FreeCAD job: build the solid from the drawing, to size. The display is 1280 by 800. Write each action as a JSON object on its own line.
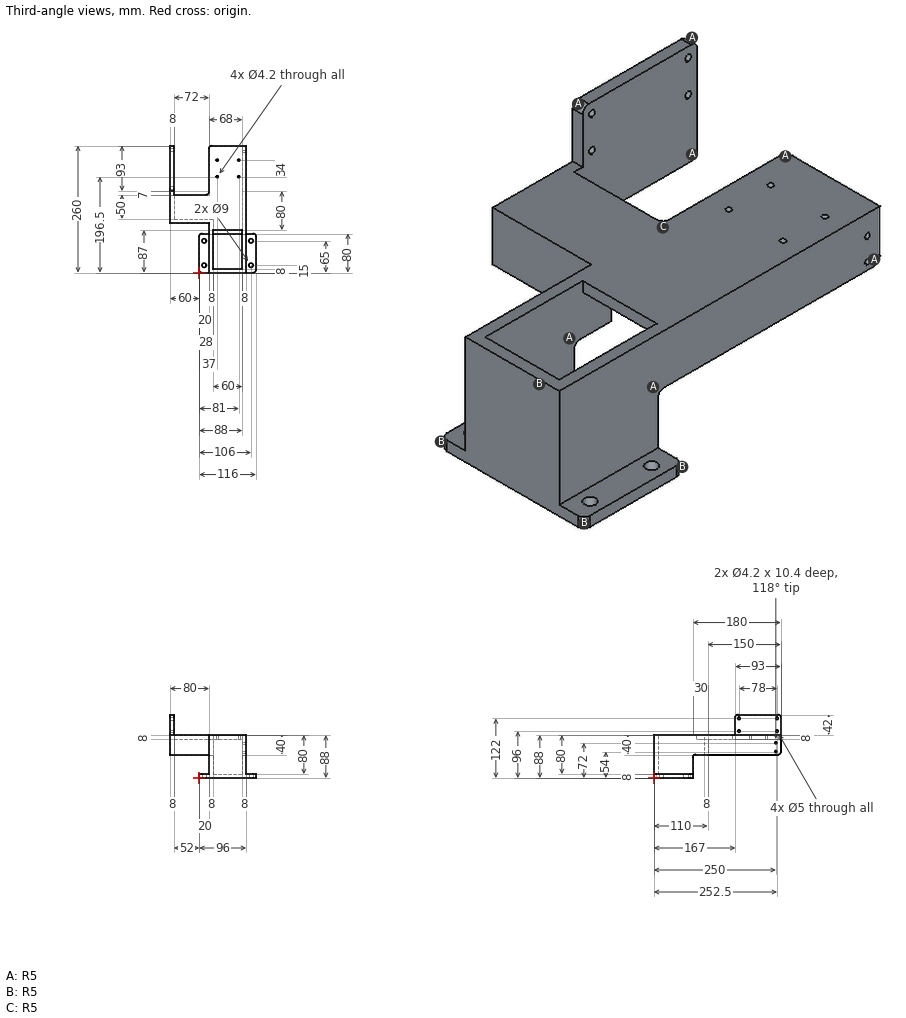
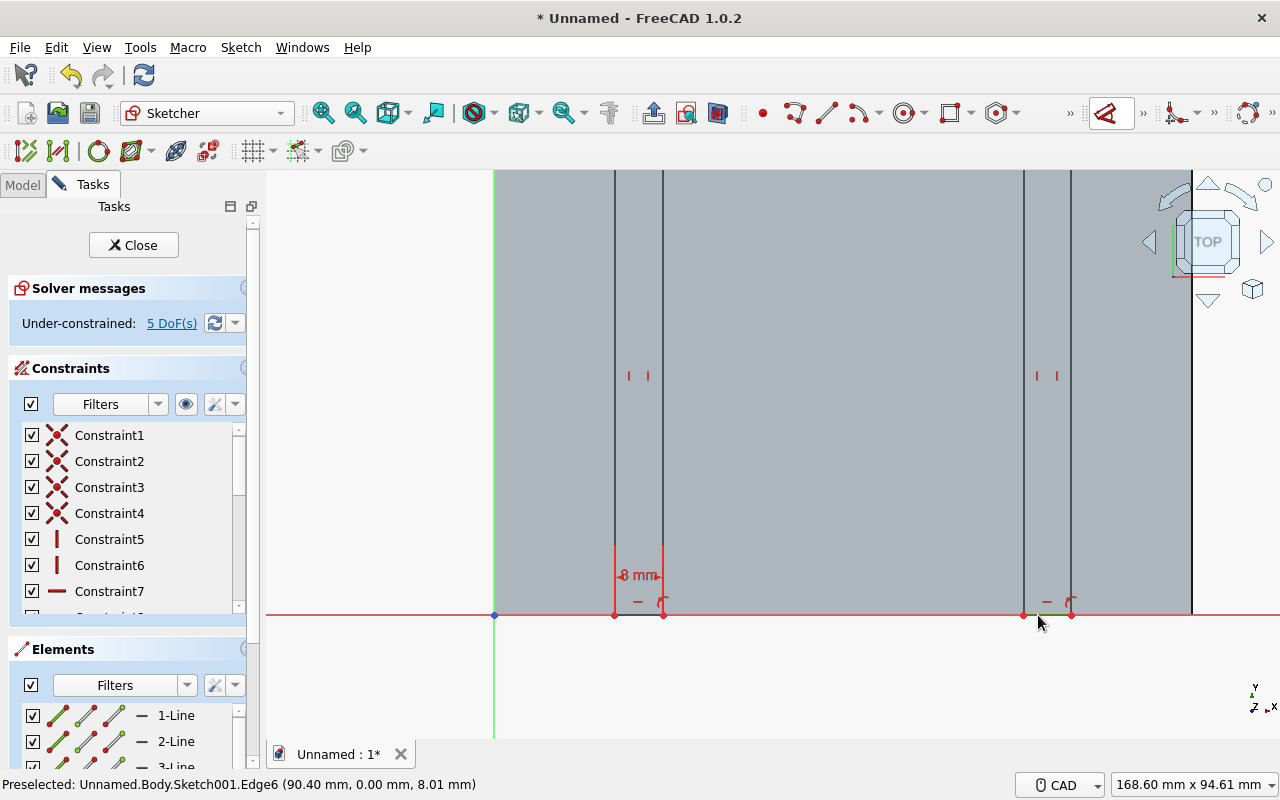
{"action": "left_click", "coordinate": [1128, 114]}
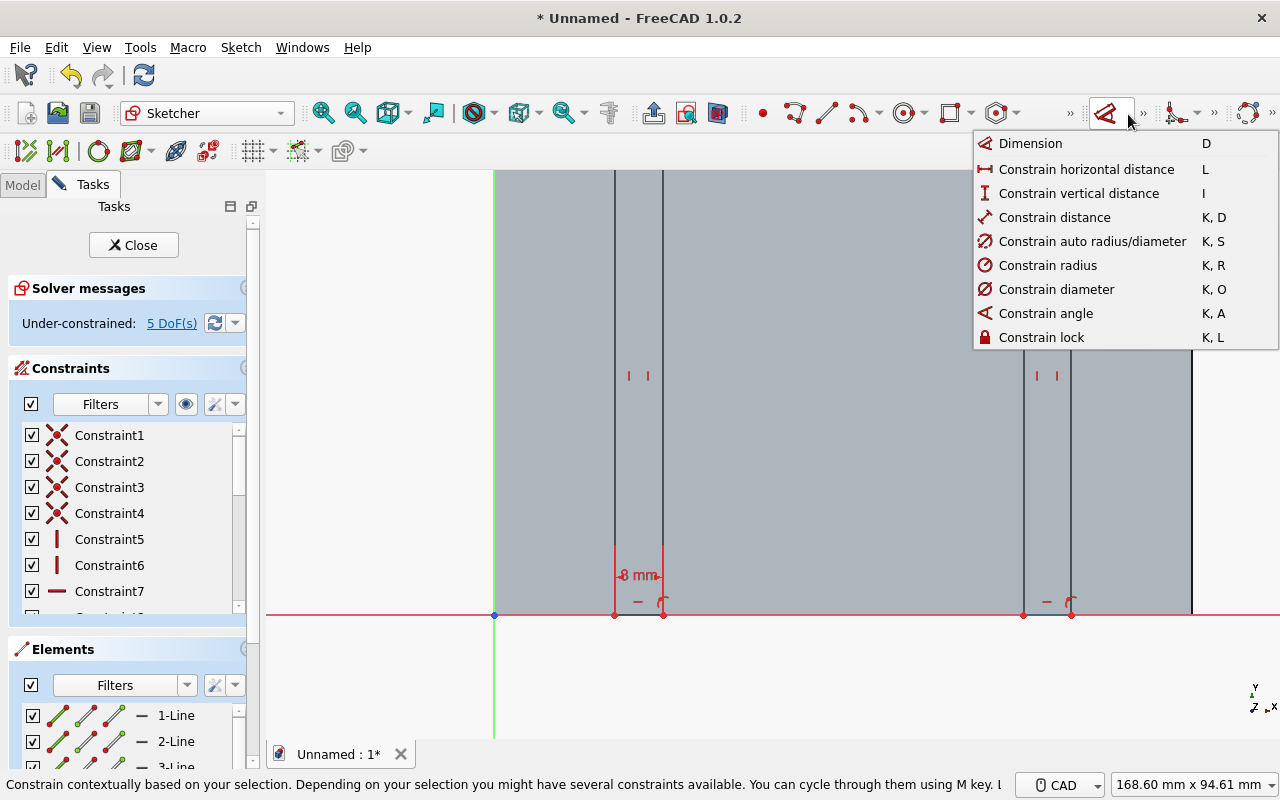
{"action": "left_click", "coordinate": [1126, 169]}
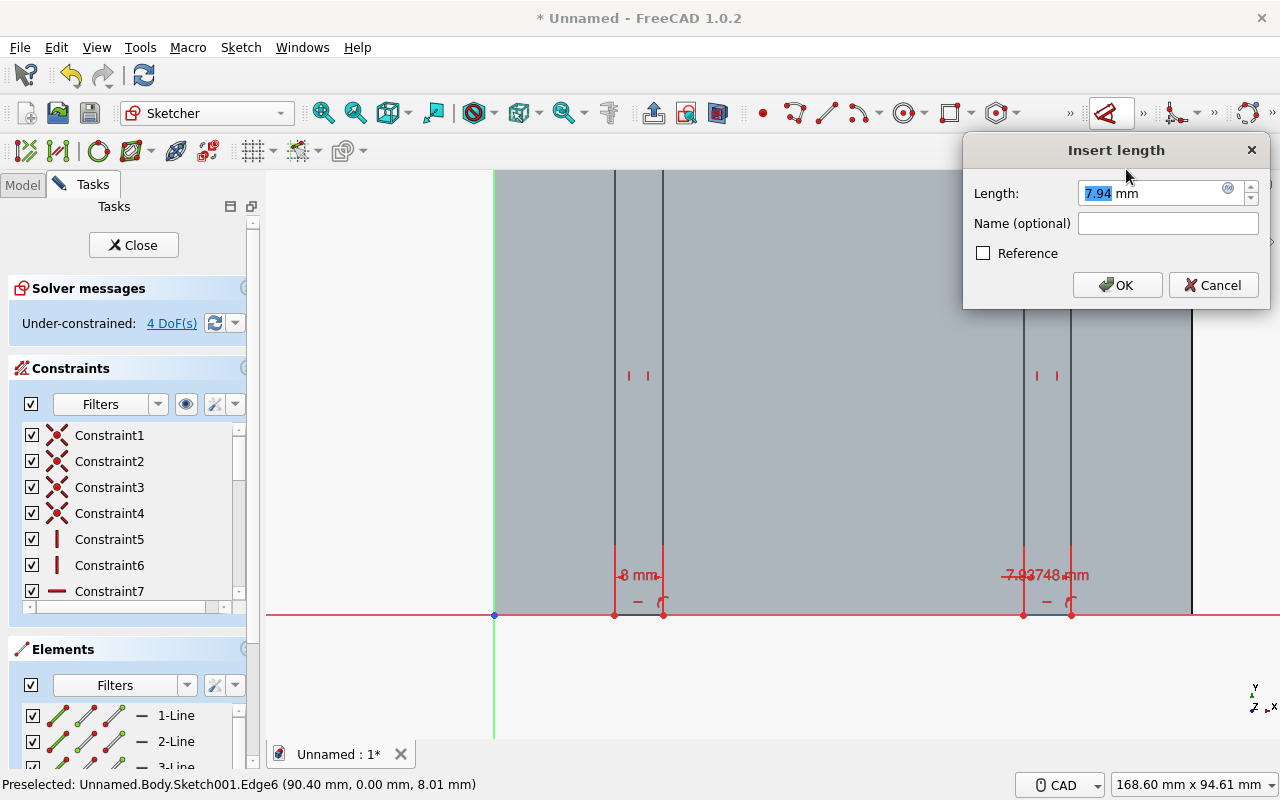
{"action": "type", "text": "8"}
{"action": "key", "text": "Return"}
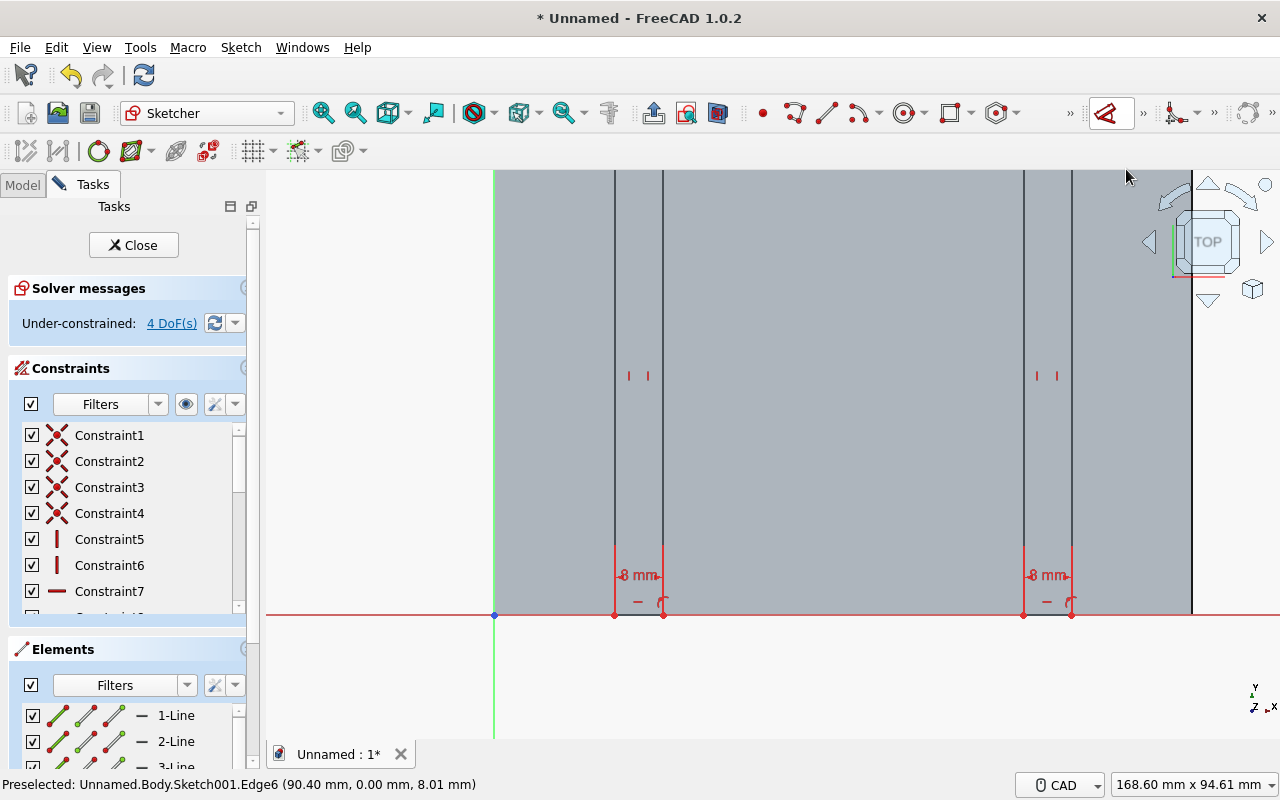
{"action": "left_click", "coordinate": [615, 279]}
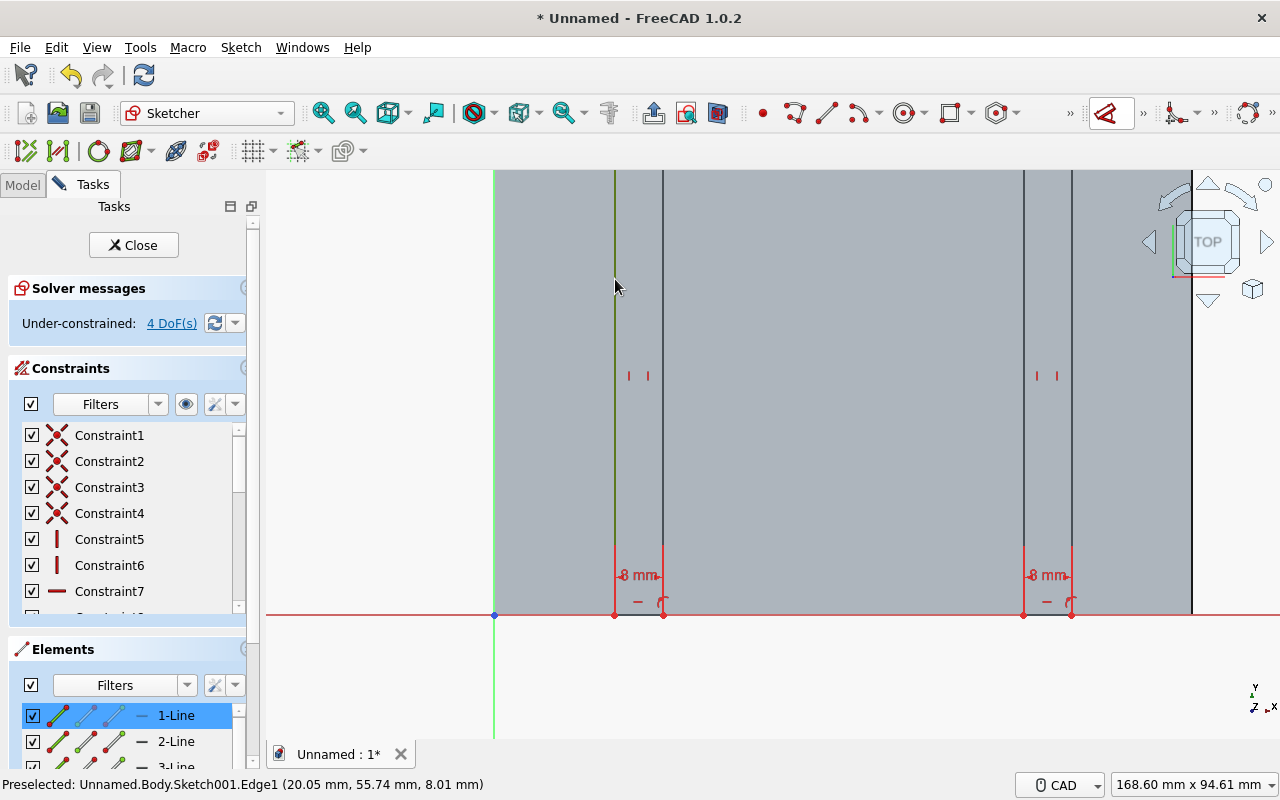
{"action": "left_click", "coordinate": [1128, 114]}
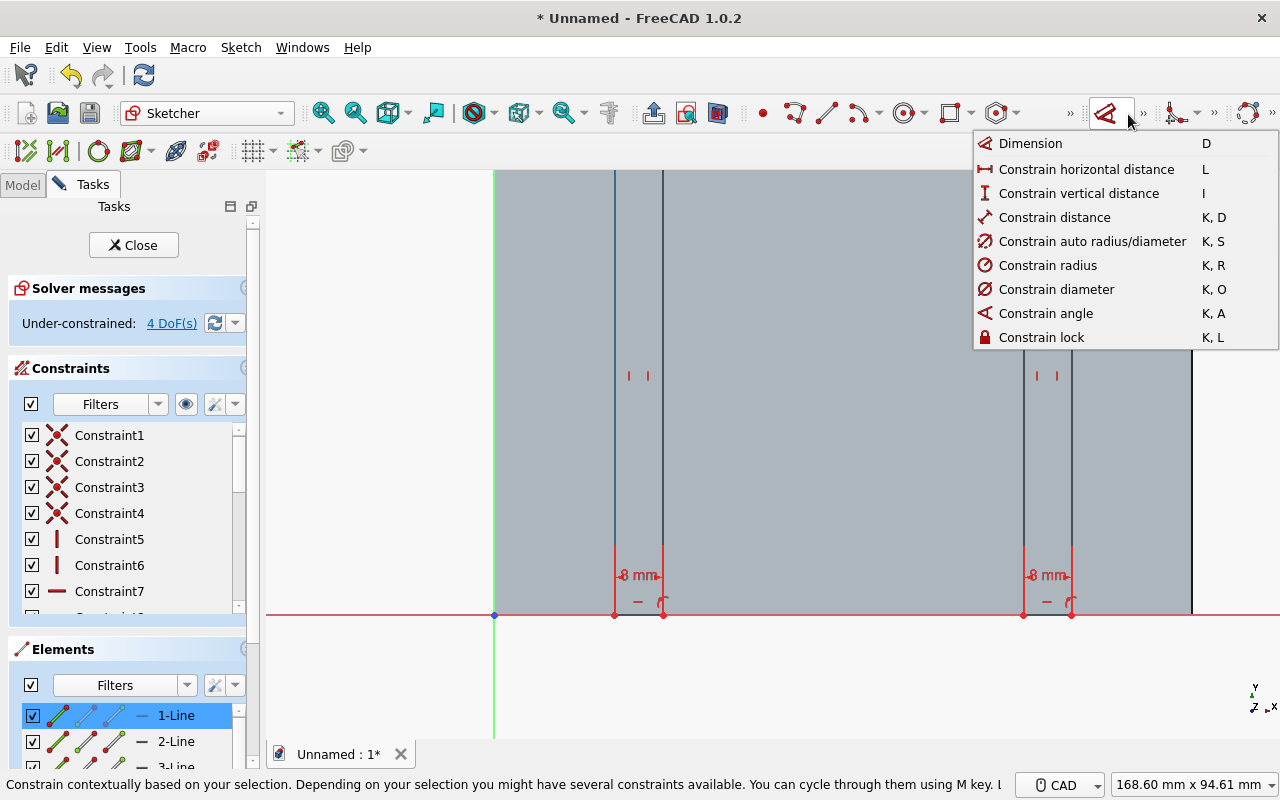
{"action": "left_click", "coordinate": [1126, 193]}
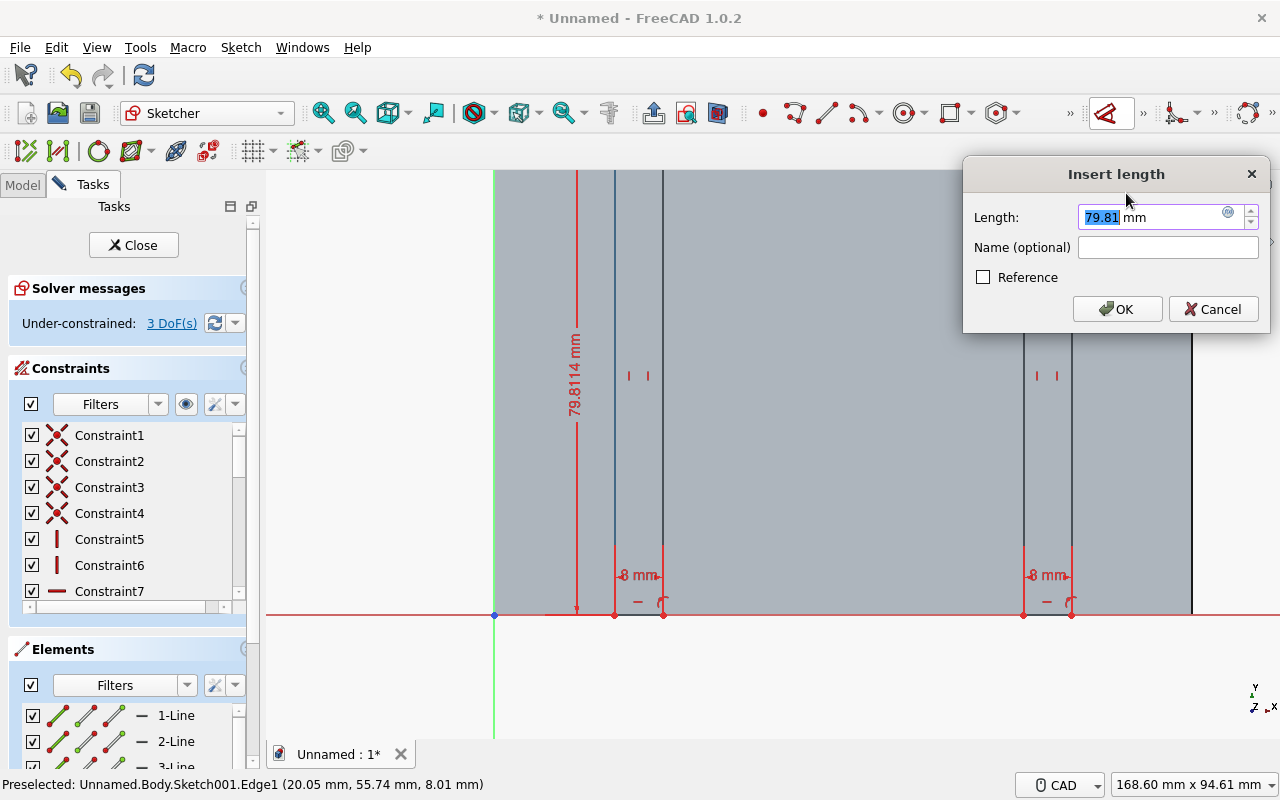
{"action": "type", "text": "80"}
{"action": "key", "text": "Return"}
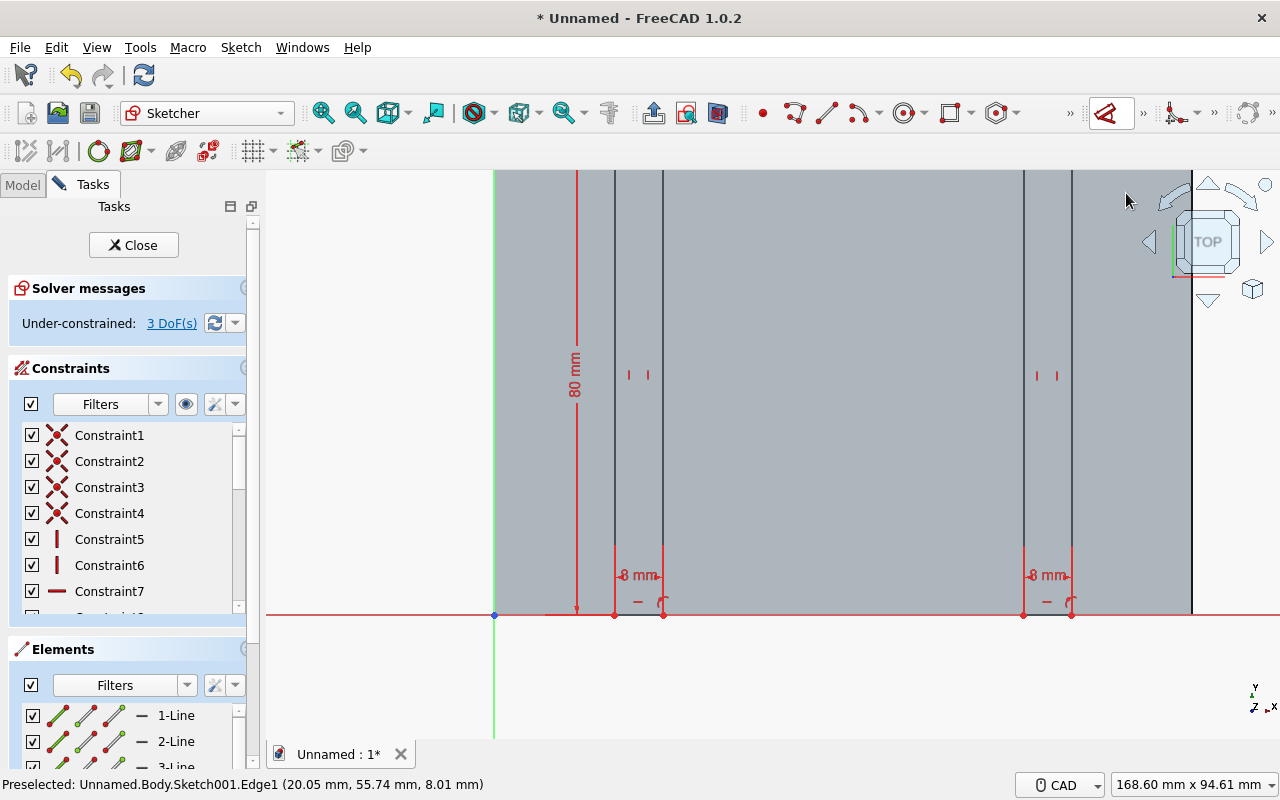
{"action": "left_click", "coordinate": [1024, 279]}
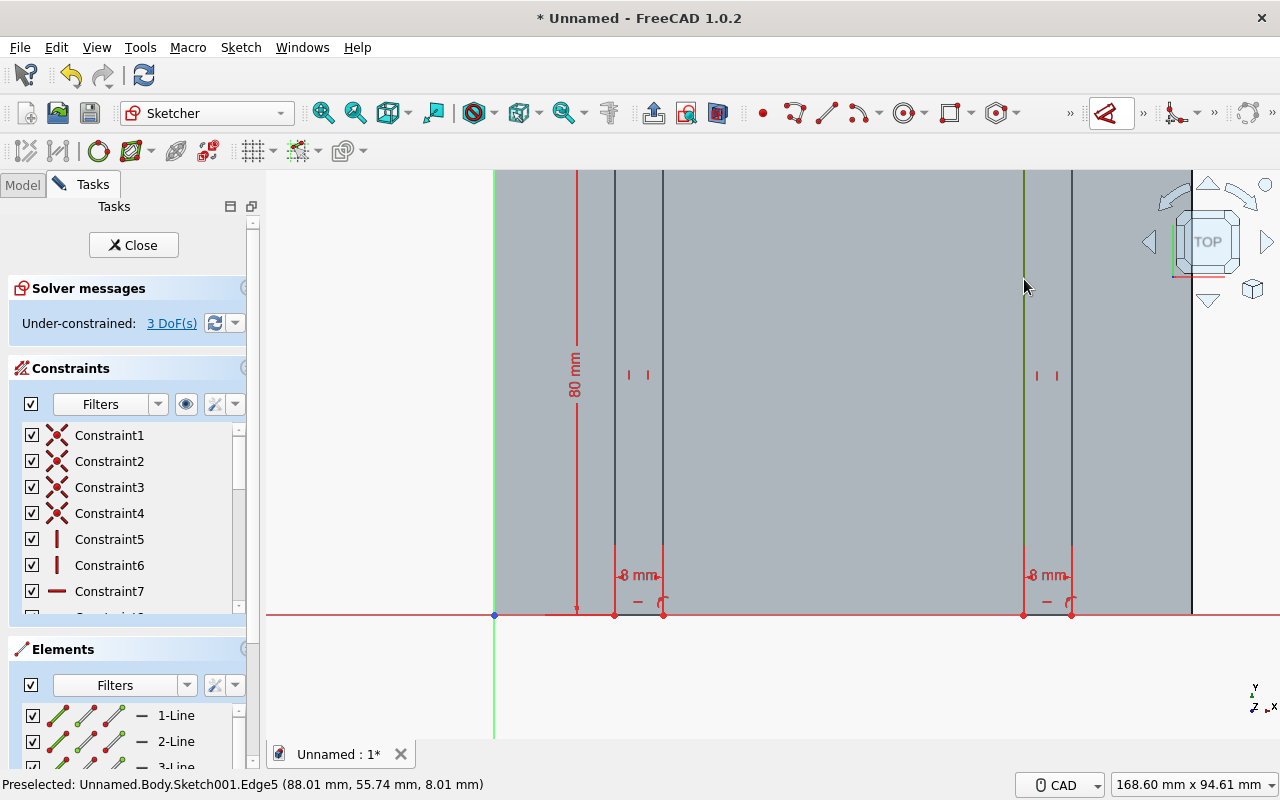
{"action": "key", "text": "i"}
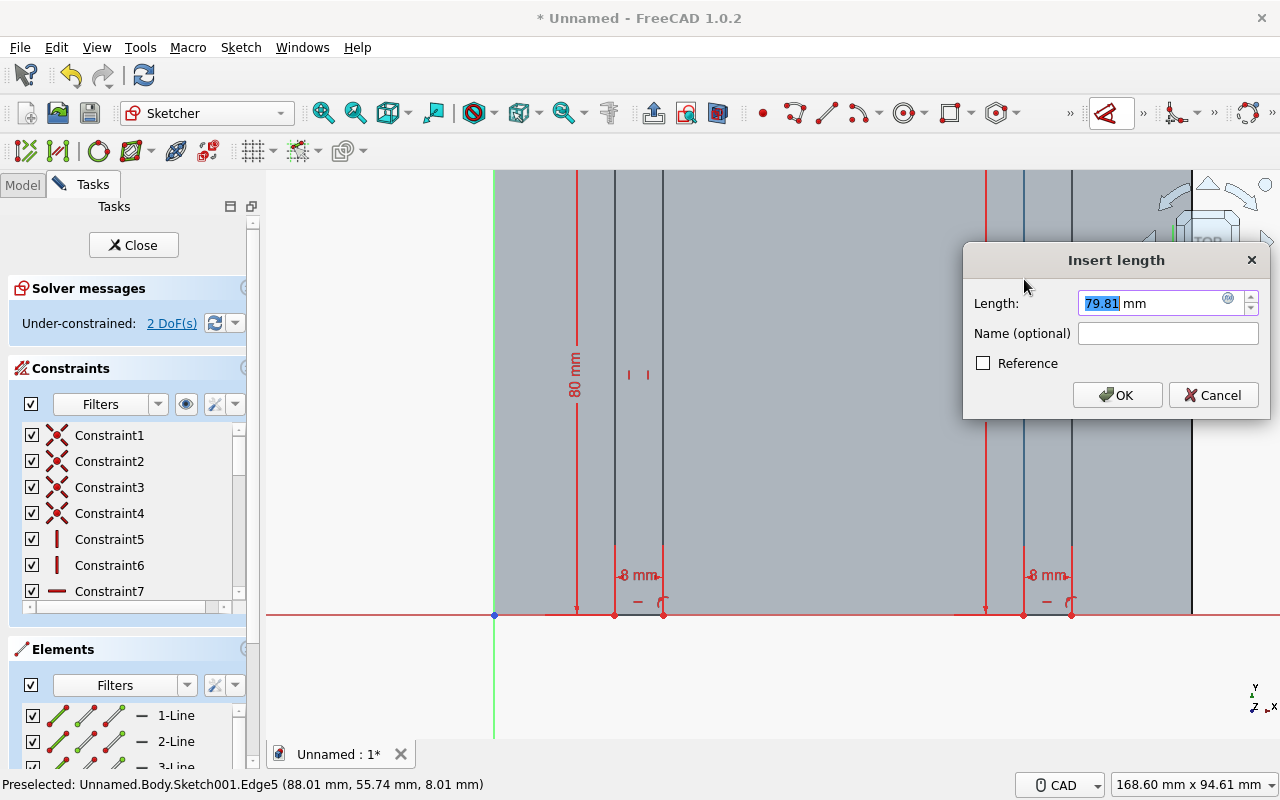
{"action": "type", "text": "80"}
{"action": "key", "text": "Return"}